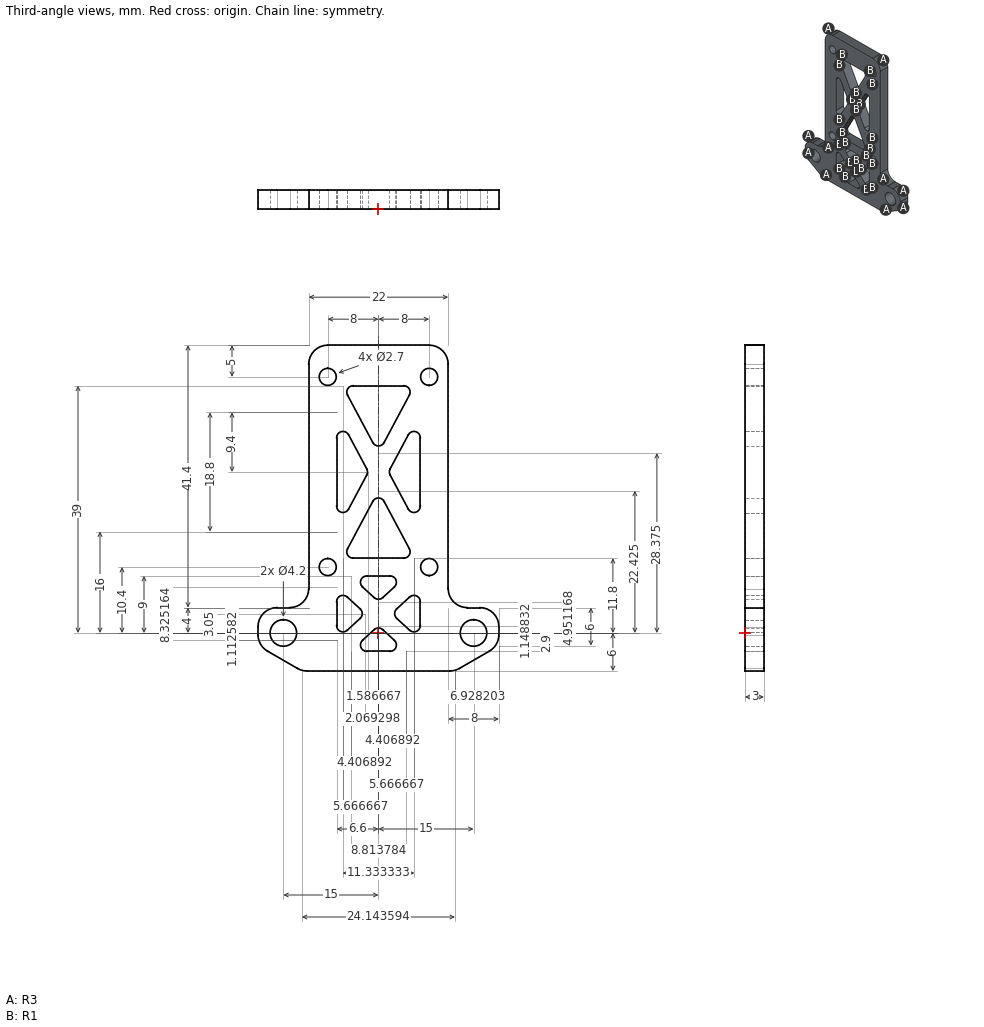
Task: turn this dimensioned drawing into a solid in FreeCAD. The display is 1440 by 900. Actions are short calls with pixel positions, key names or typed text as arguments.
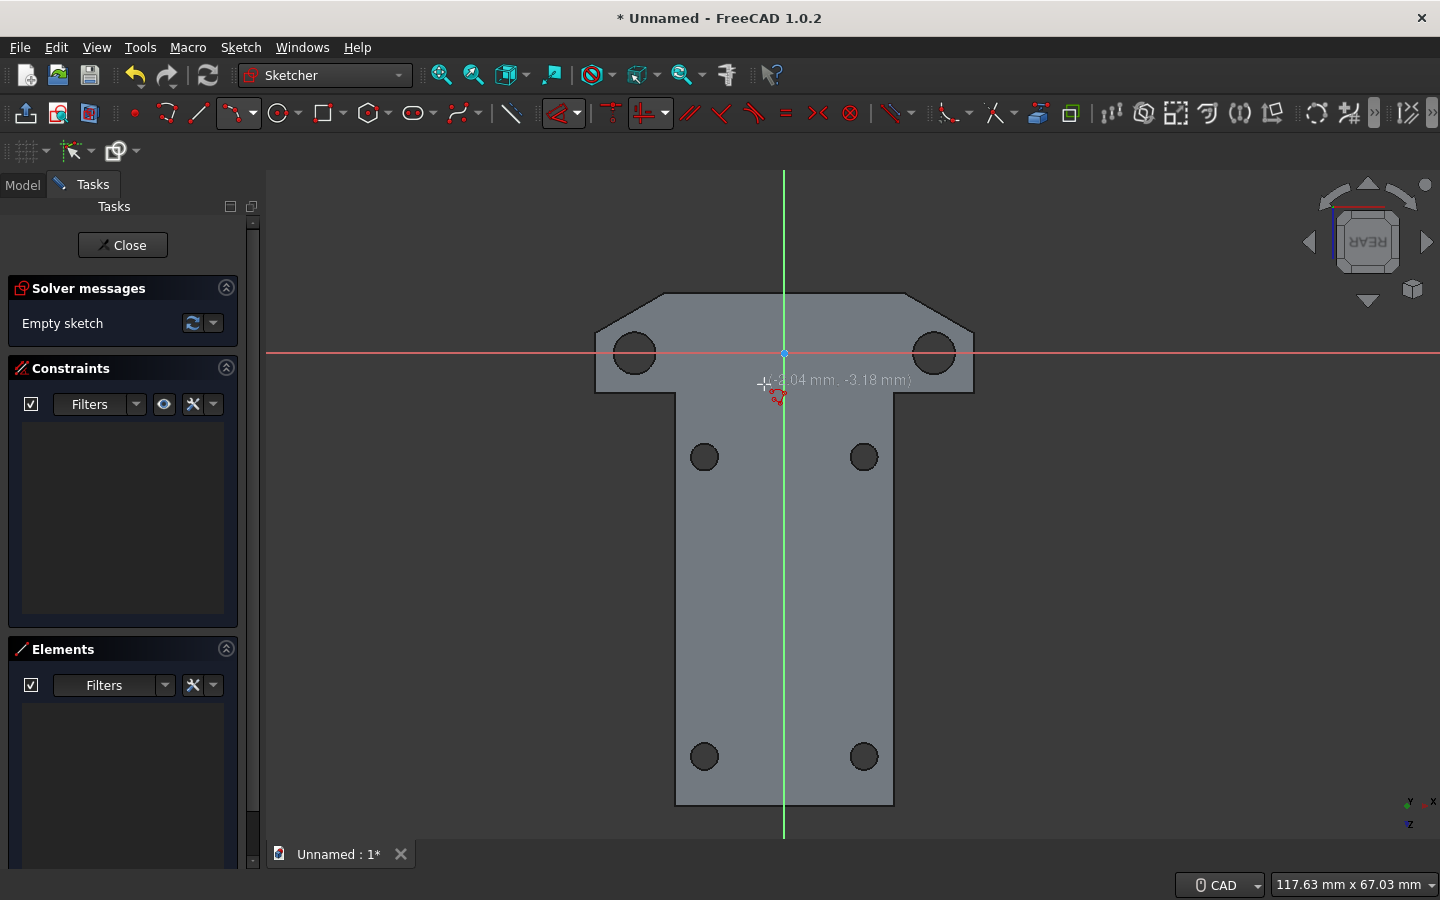
scroll(718, 342, up, 2)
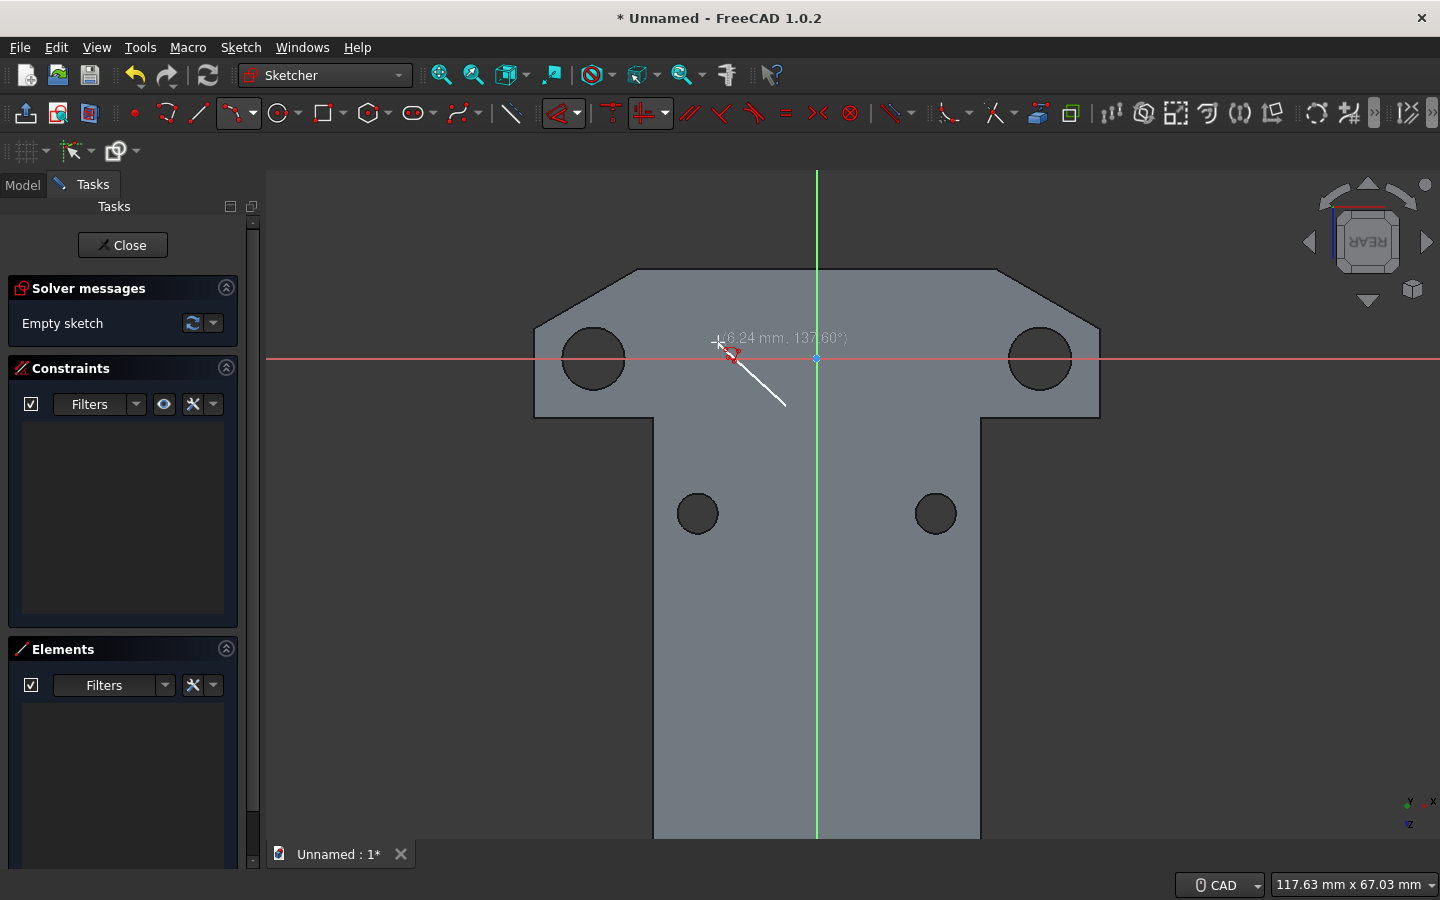
click(718, 342)
click(718, 466)
click(786, 406)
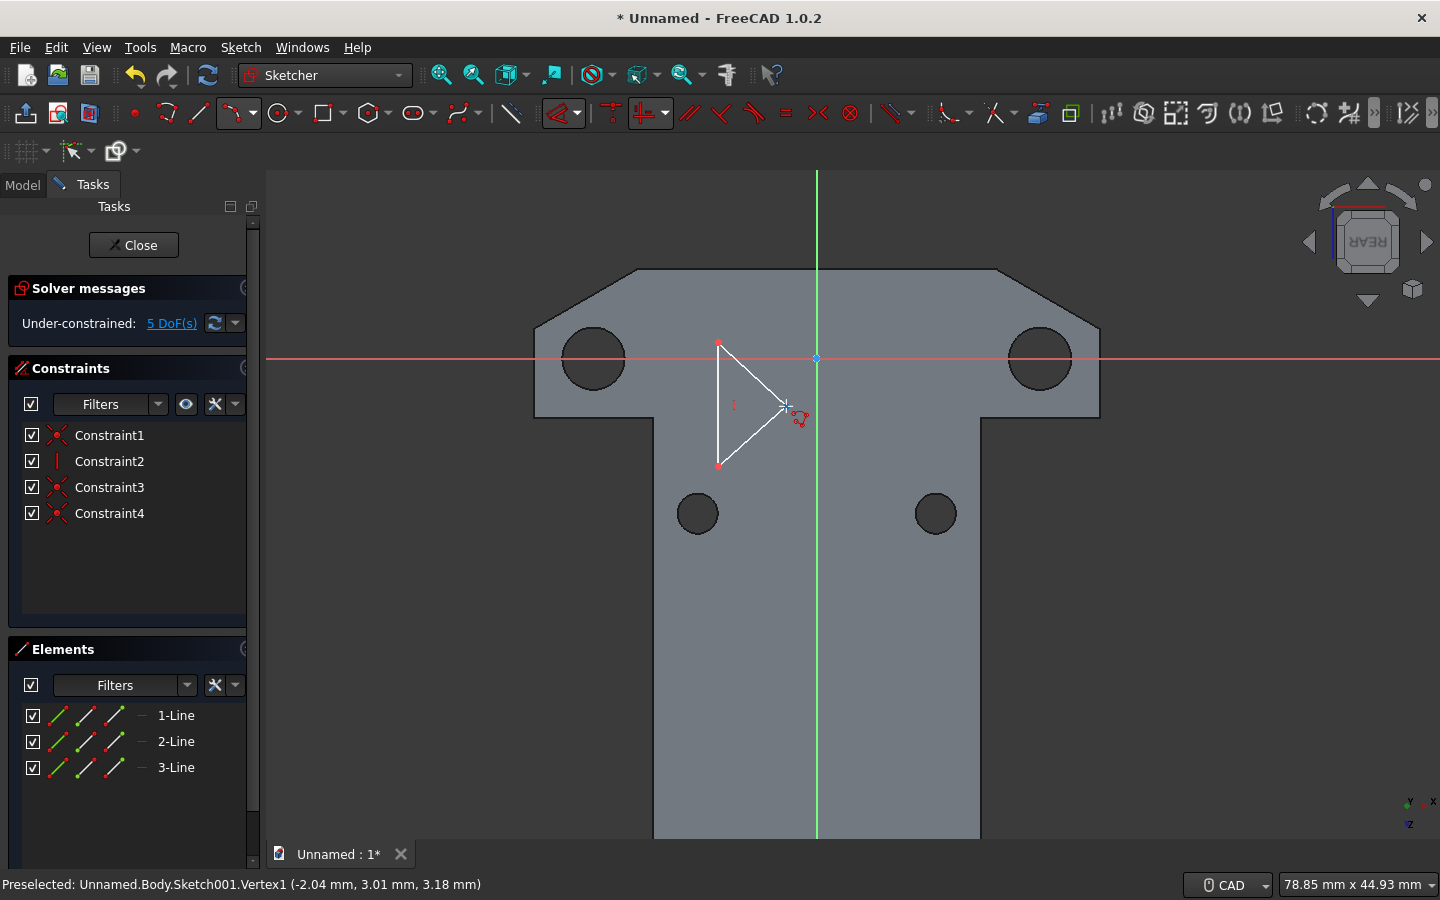
click(817, 376)
click(882, 316)
click(751, 316)
click(817, 377)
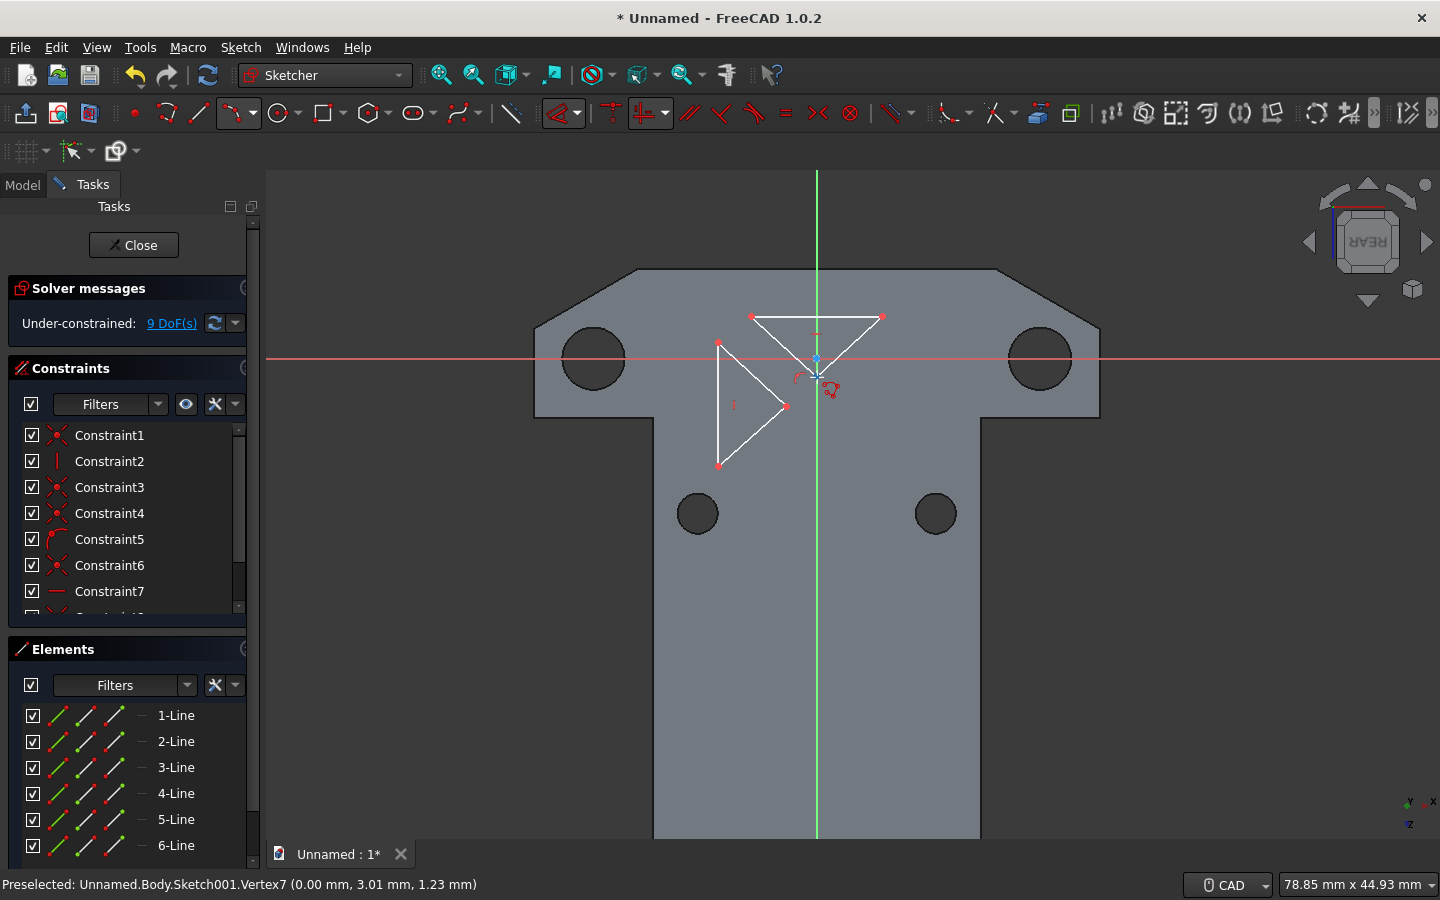
click(848, 404)
click(915, 466)
click(915, 342)
click(848, 405)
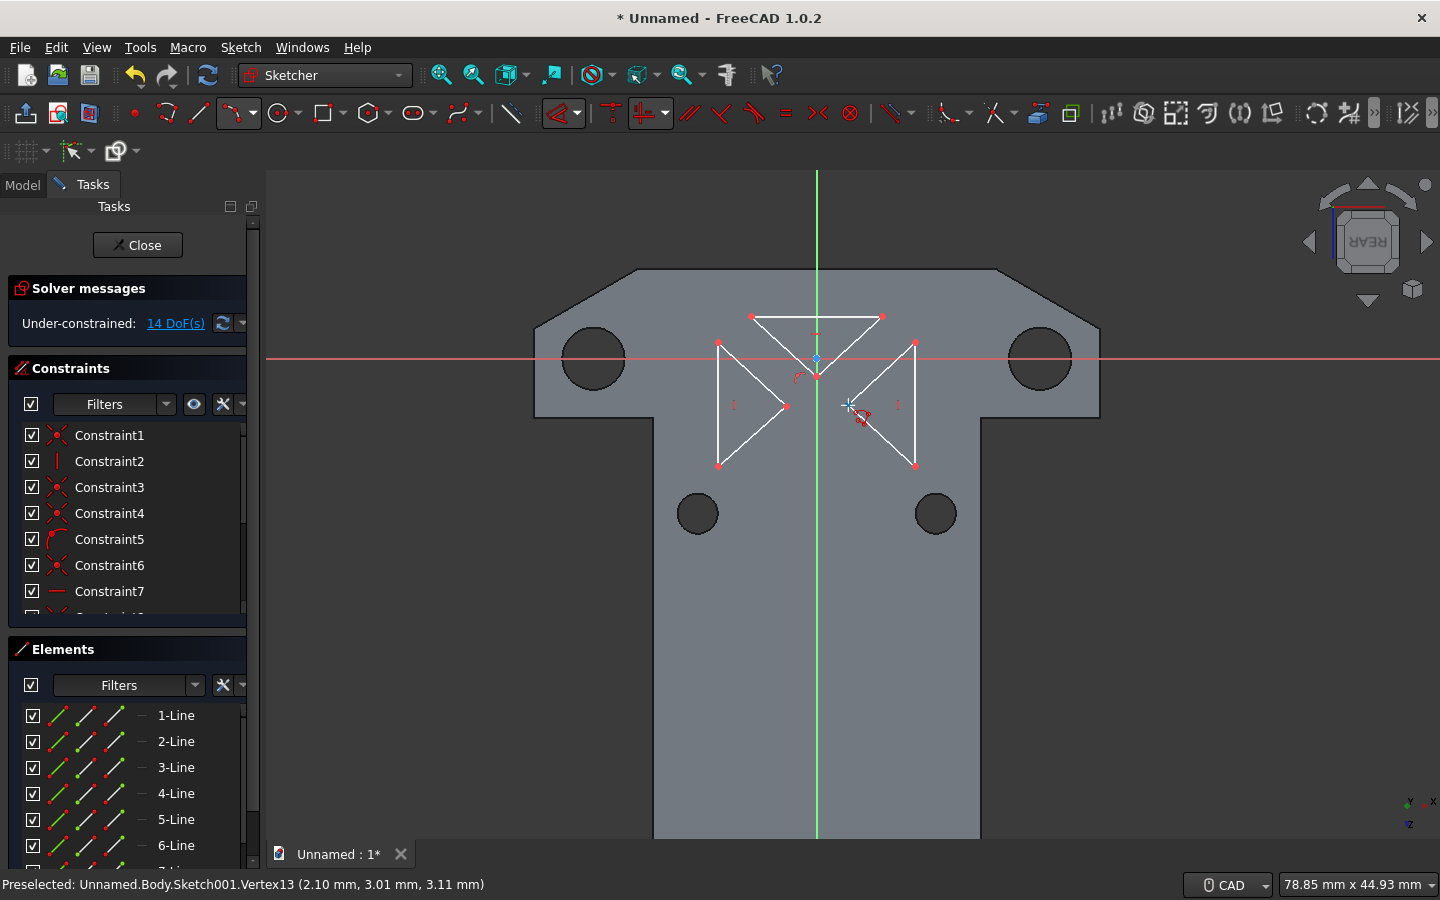
click(817, 432)
click(751, 493)
click(882, 493)
click(817, 433)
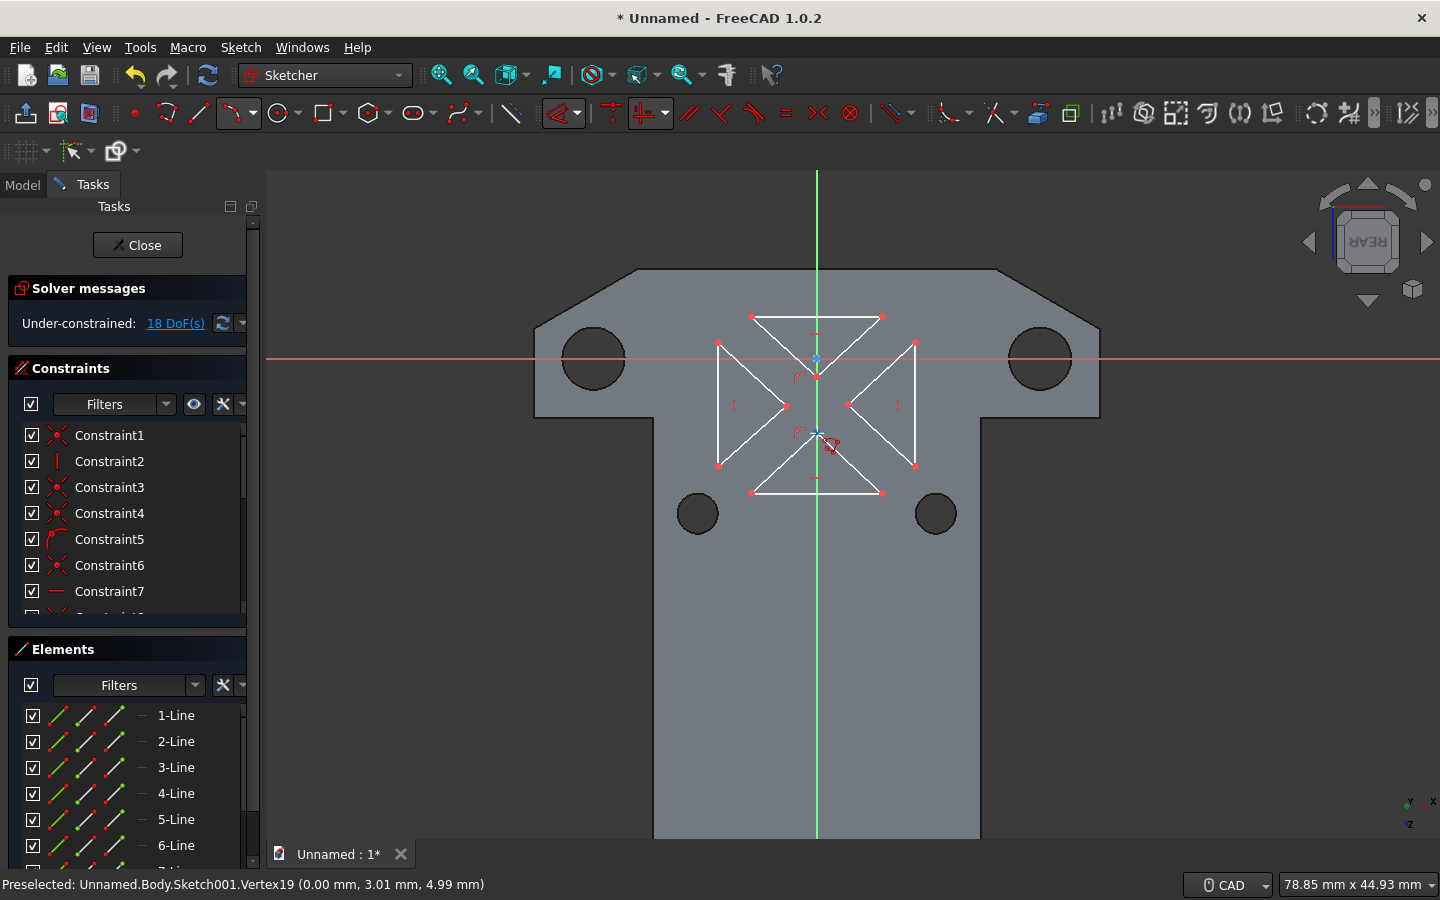
click(901, 534)
click(732, 534)
click(817, 693)
click(901, 535)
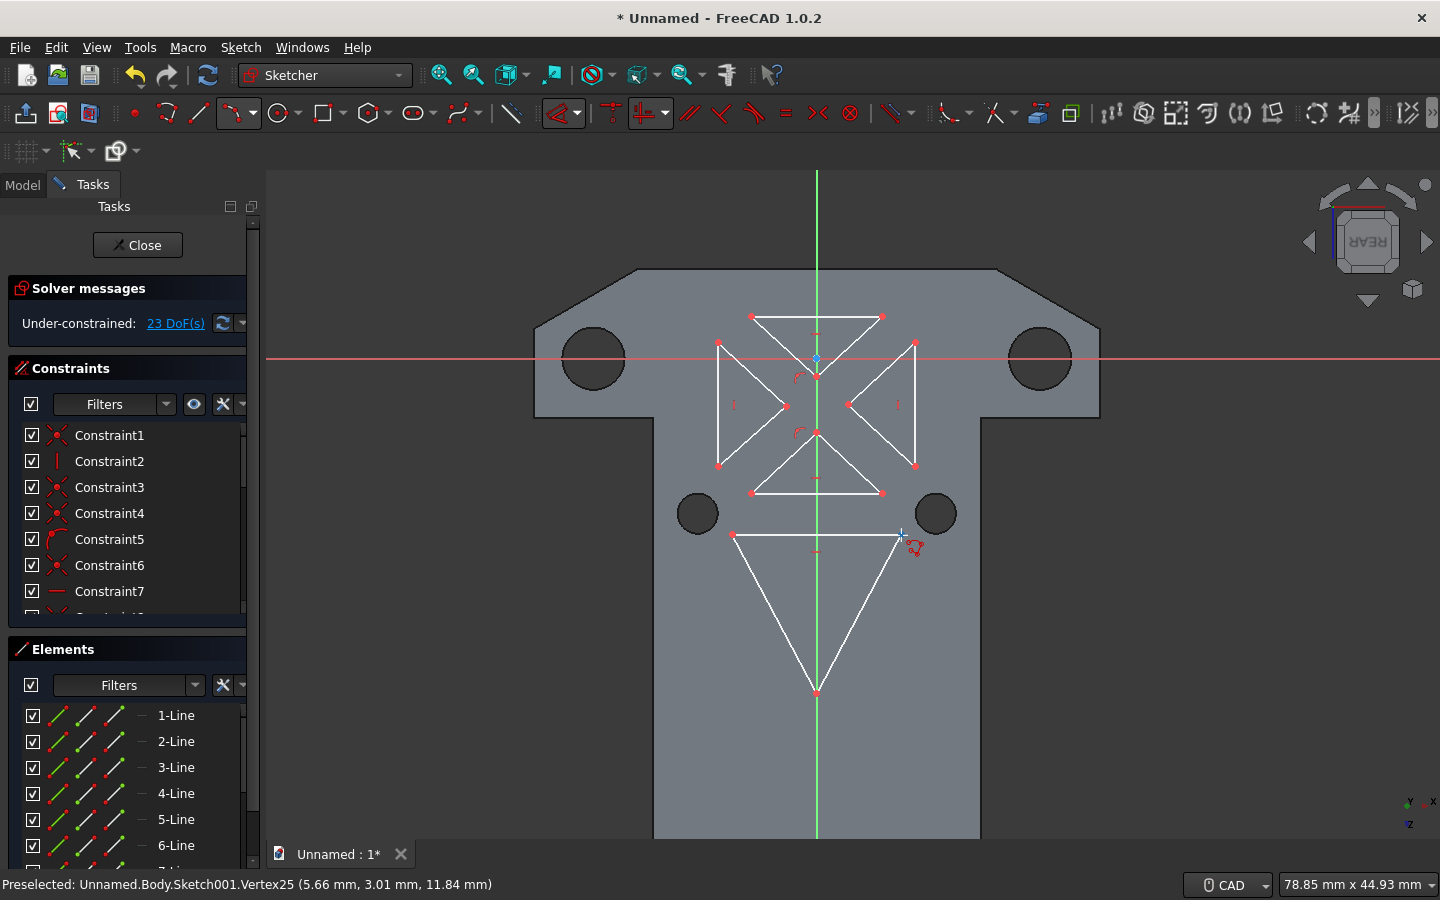
click(718, 597)